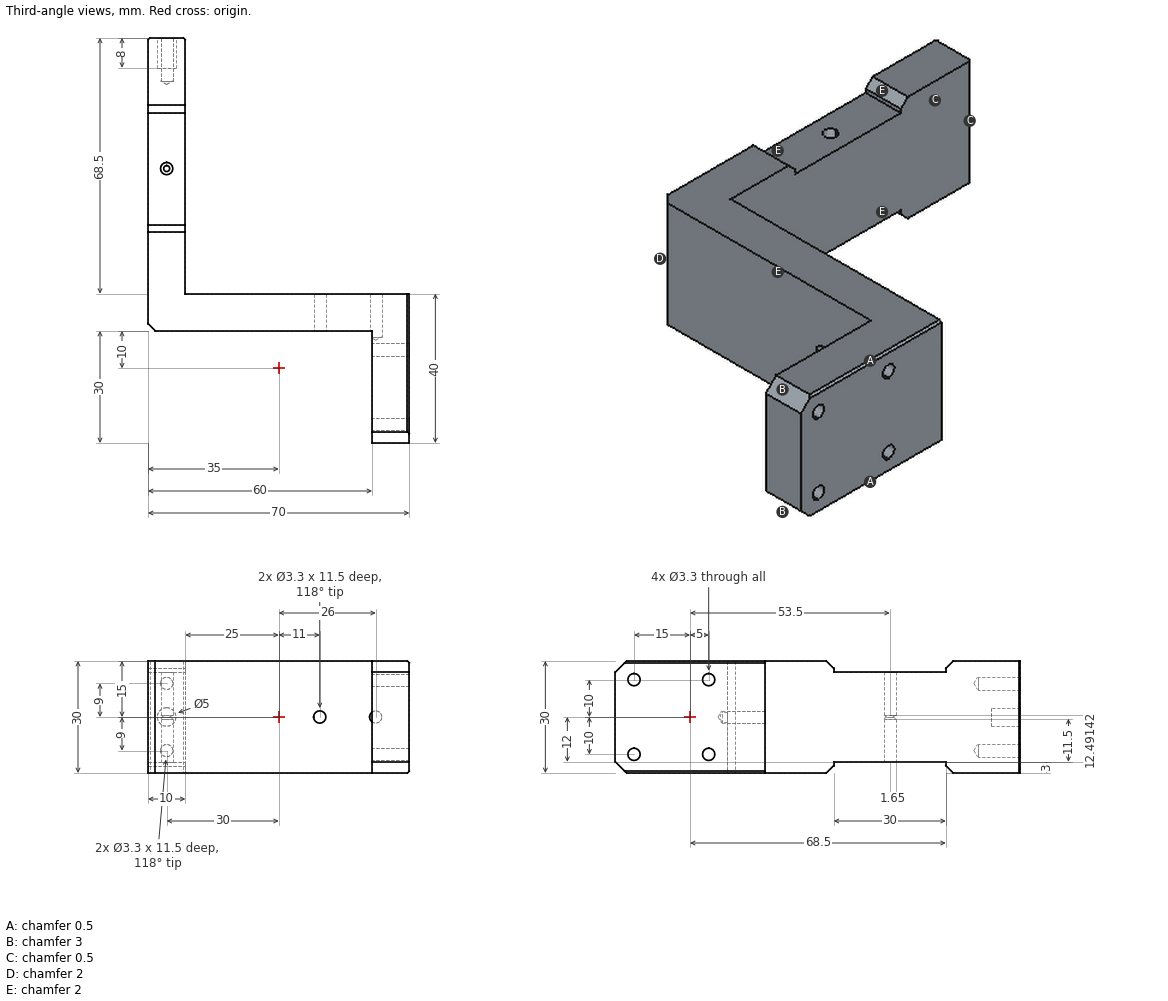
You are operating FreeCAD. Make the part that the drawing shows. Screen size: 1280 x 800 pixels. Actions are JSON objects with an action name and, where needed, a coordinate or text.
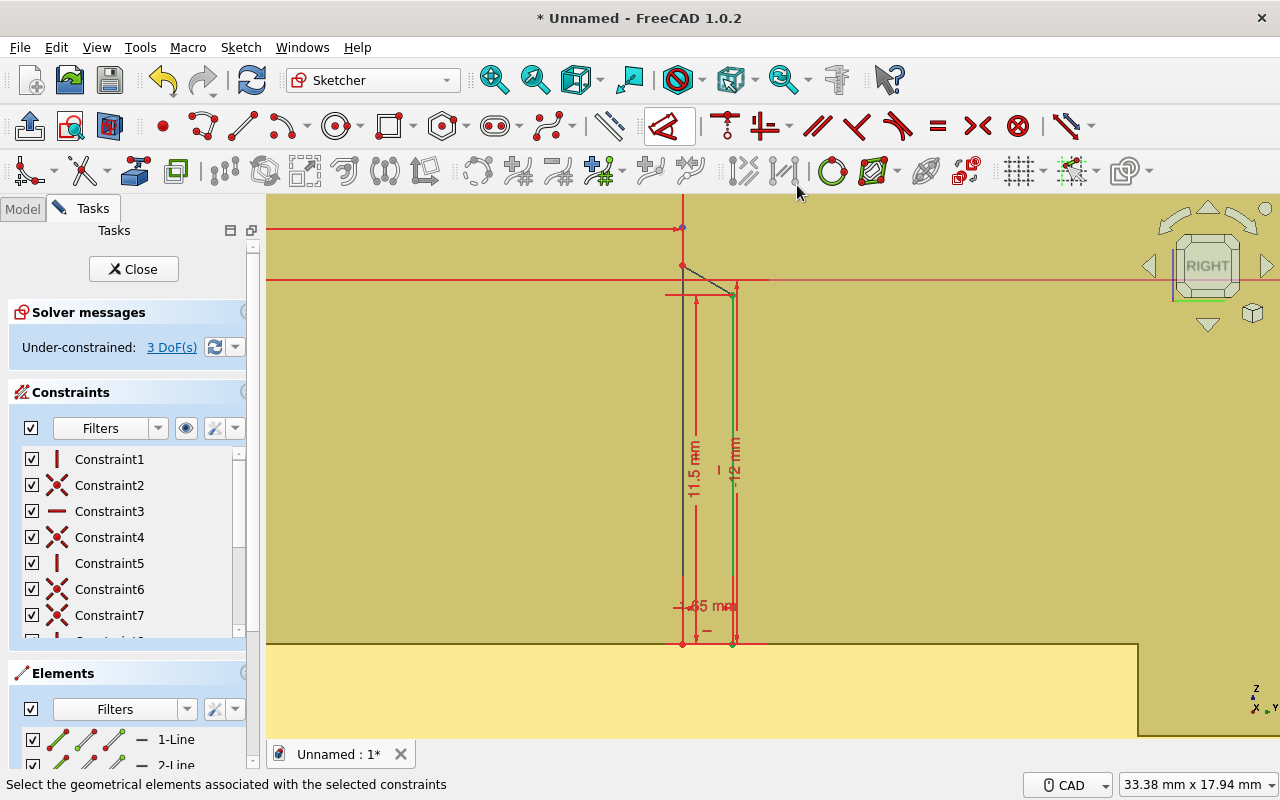
{"action": "left_click", "coordinate": [683, 379]}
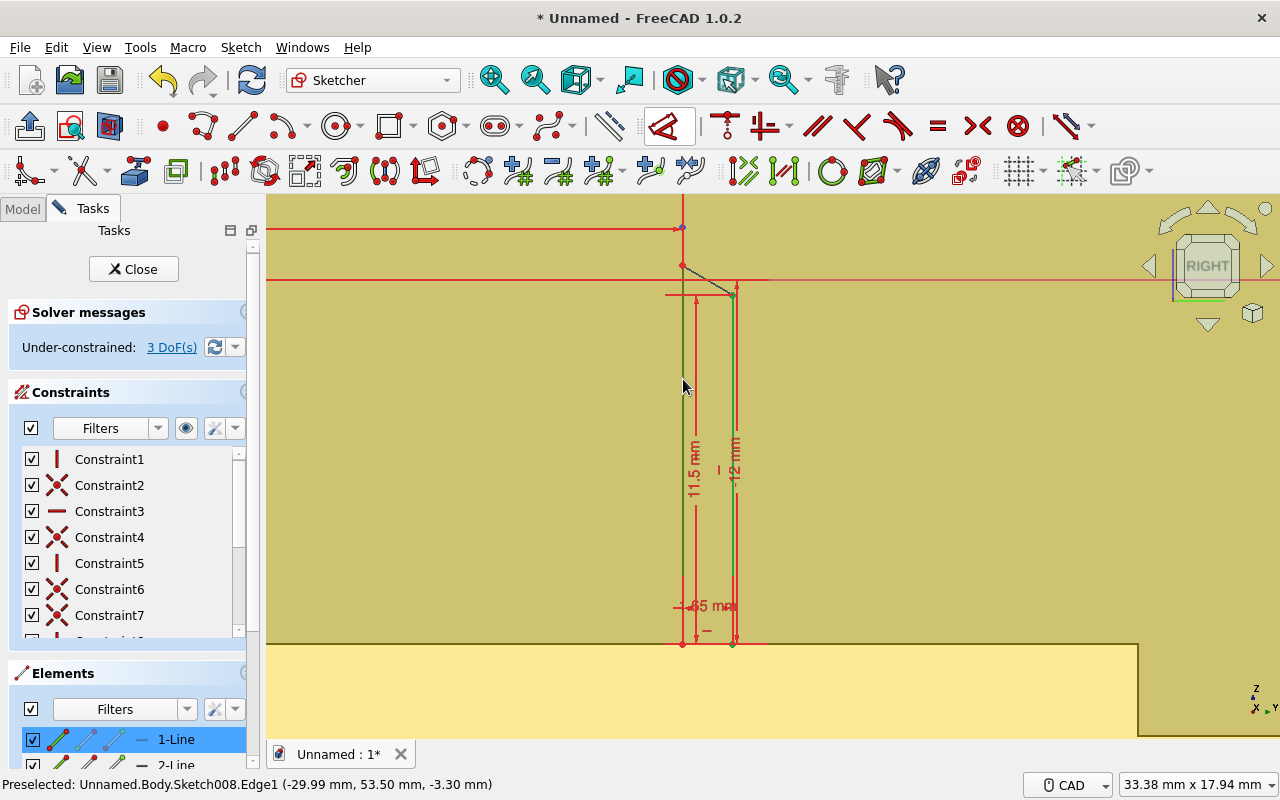
{"action": "key", "text": "i"}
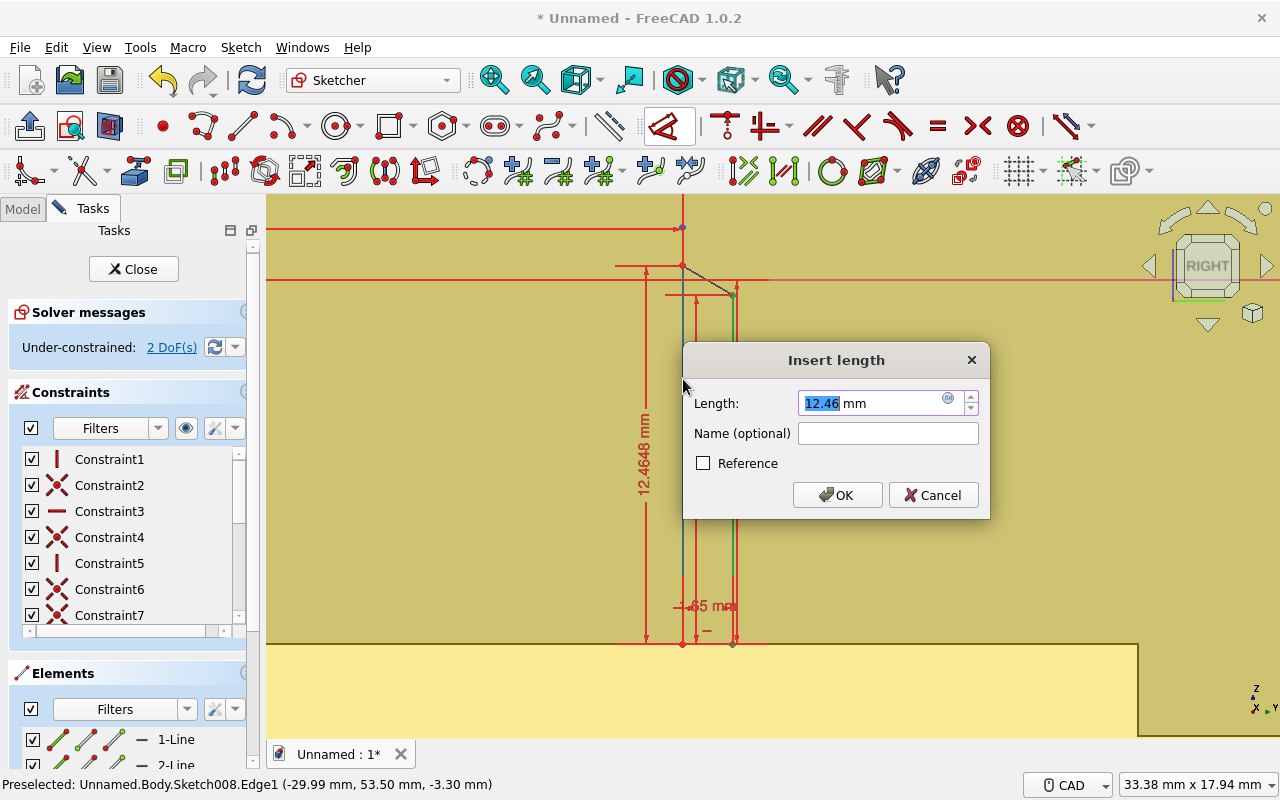
{"action": "type", "text": "12.49142"}
{"action": "key", "text": "Return"}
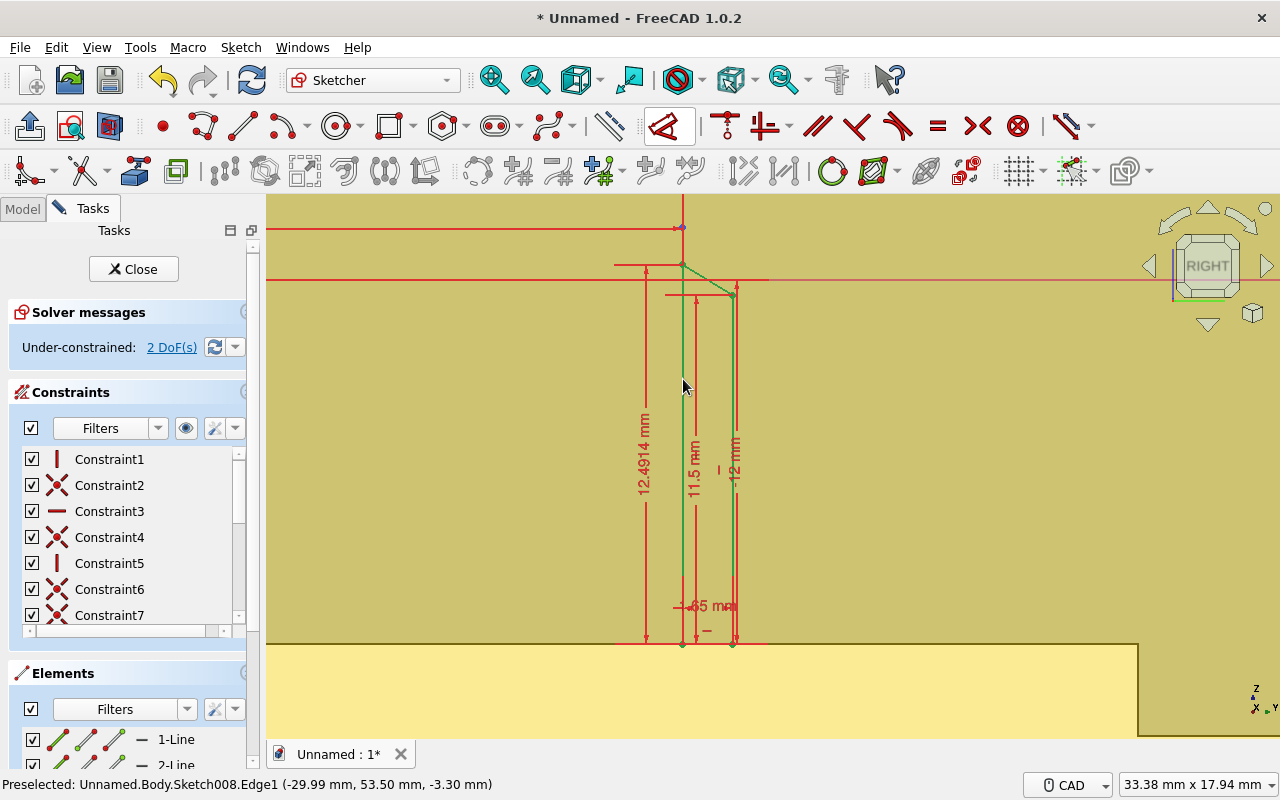
{"action": "left_click", "coordinate": [134, 269]}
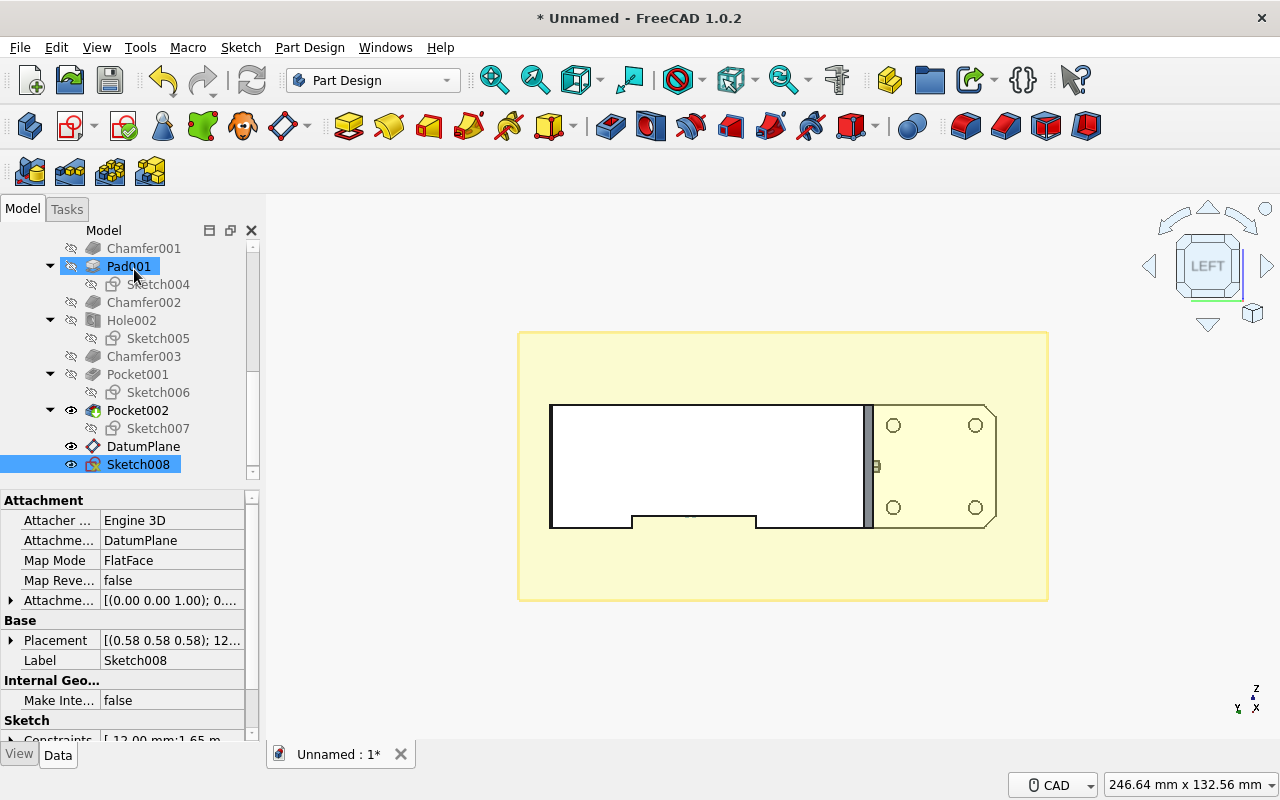
{"action": "left_click", "coordinate": [692, 126]}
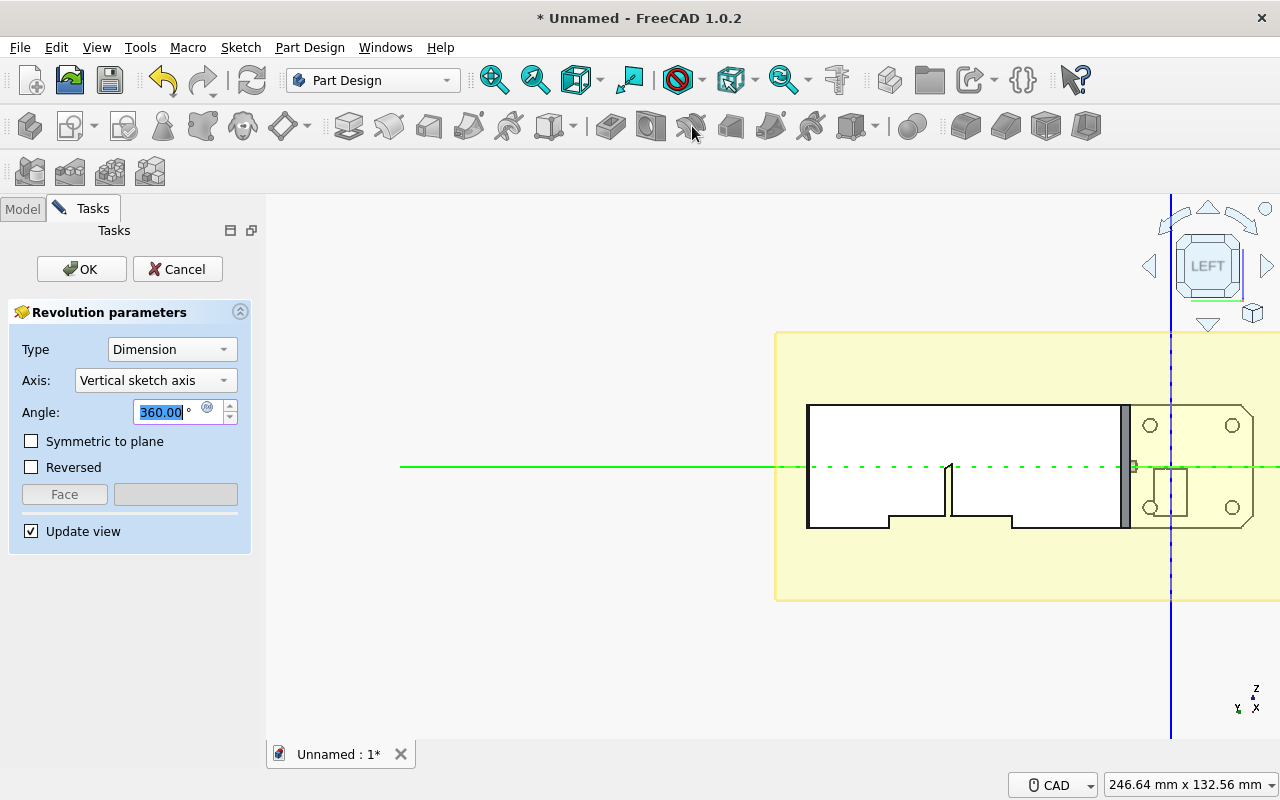
{"action": "left_click", "coordinate": [156, 380]}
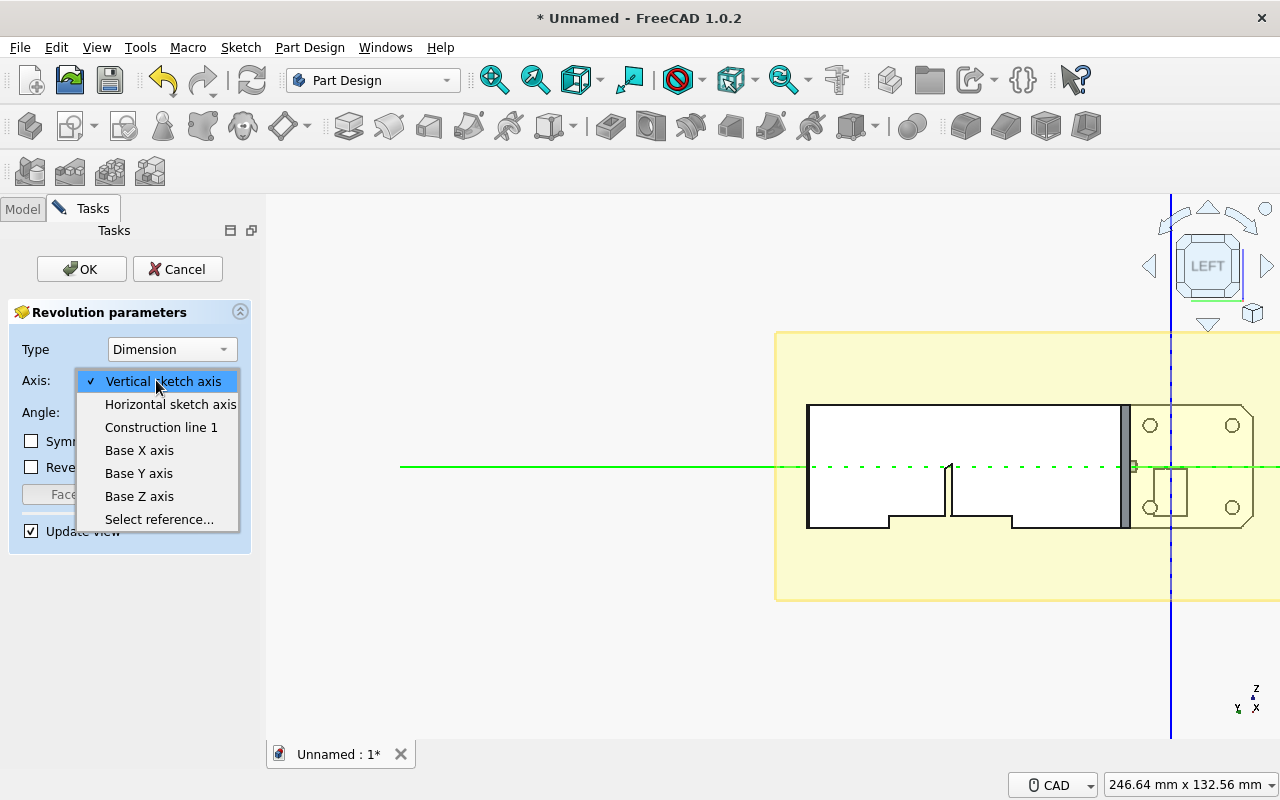
{"action": "left_click", "coordinate": [156, 428]}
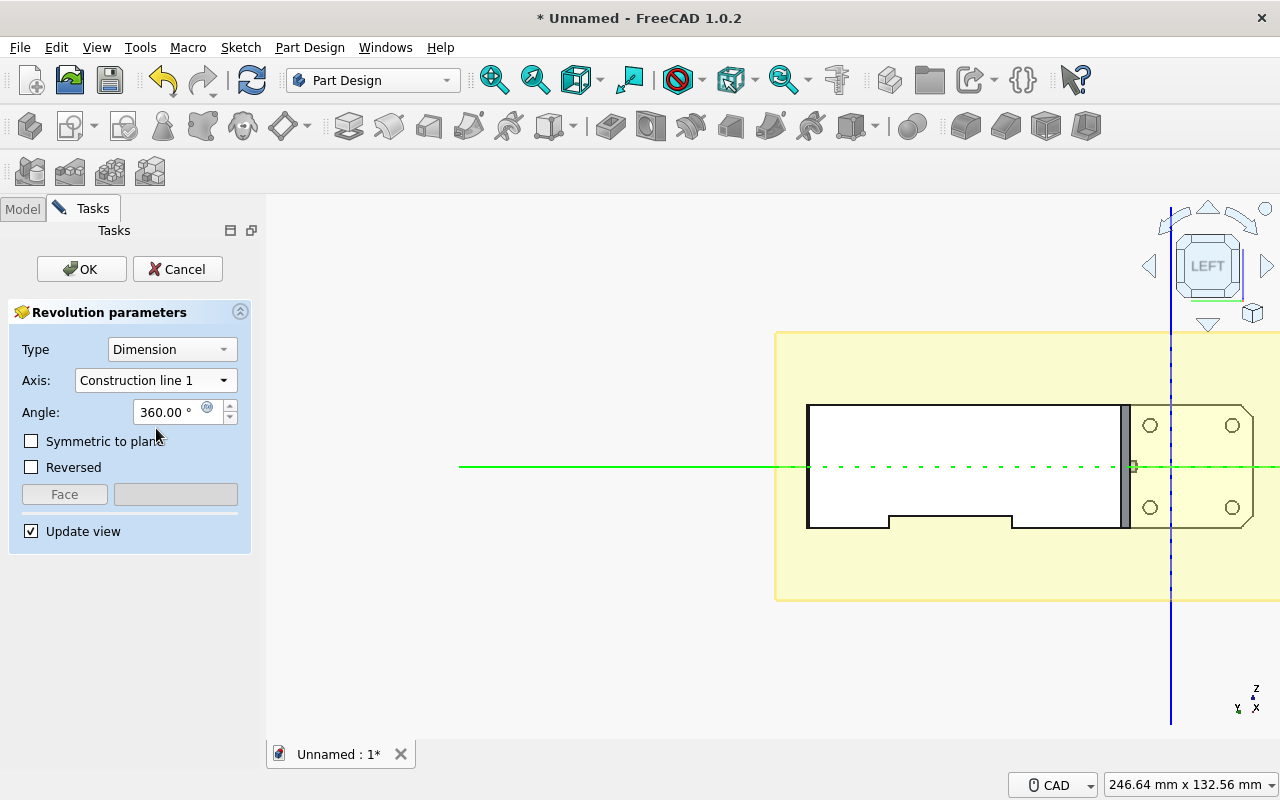
{"action": "left_click", "coordinate": [82, 269]}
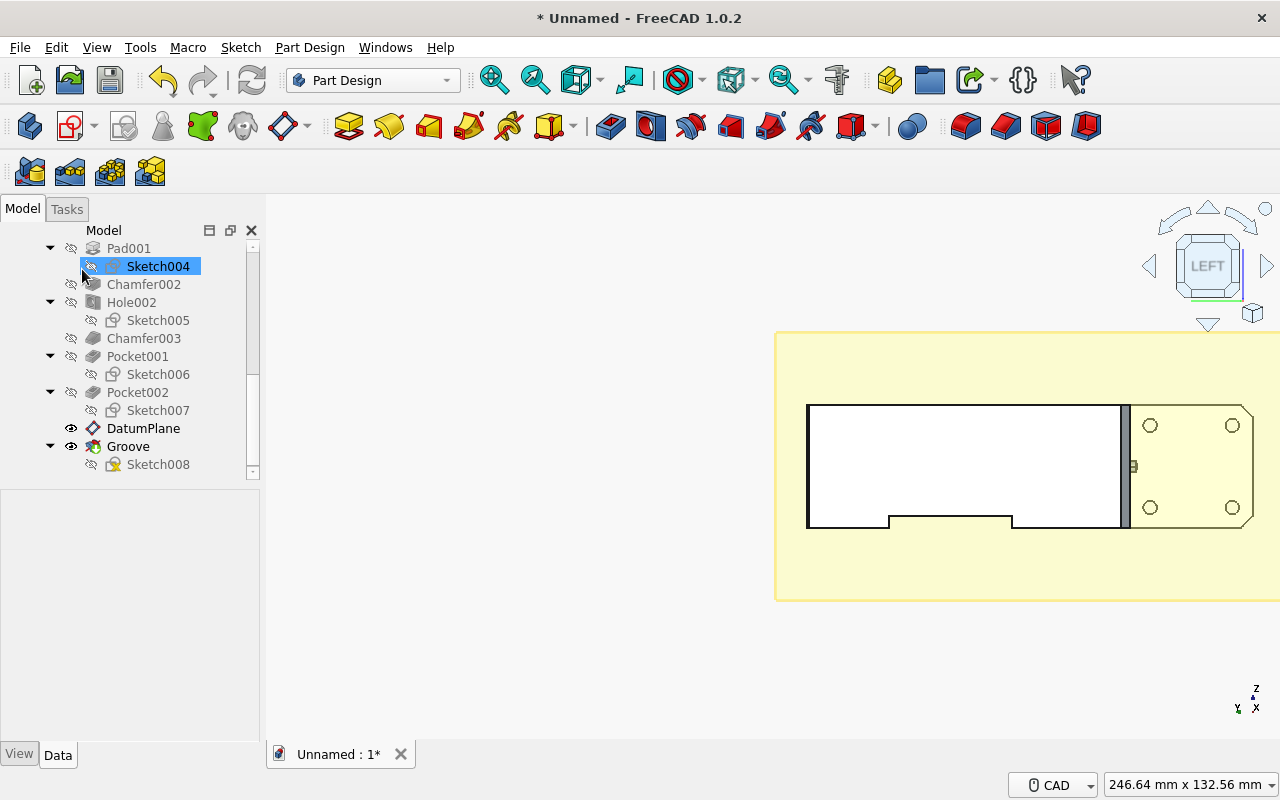
{"action": "left_click", "coordinate": [116, 428]}
{"action": "key", "text": "space"}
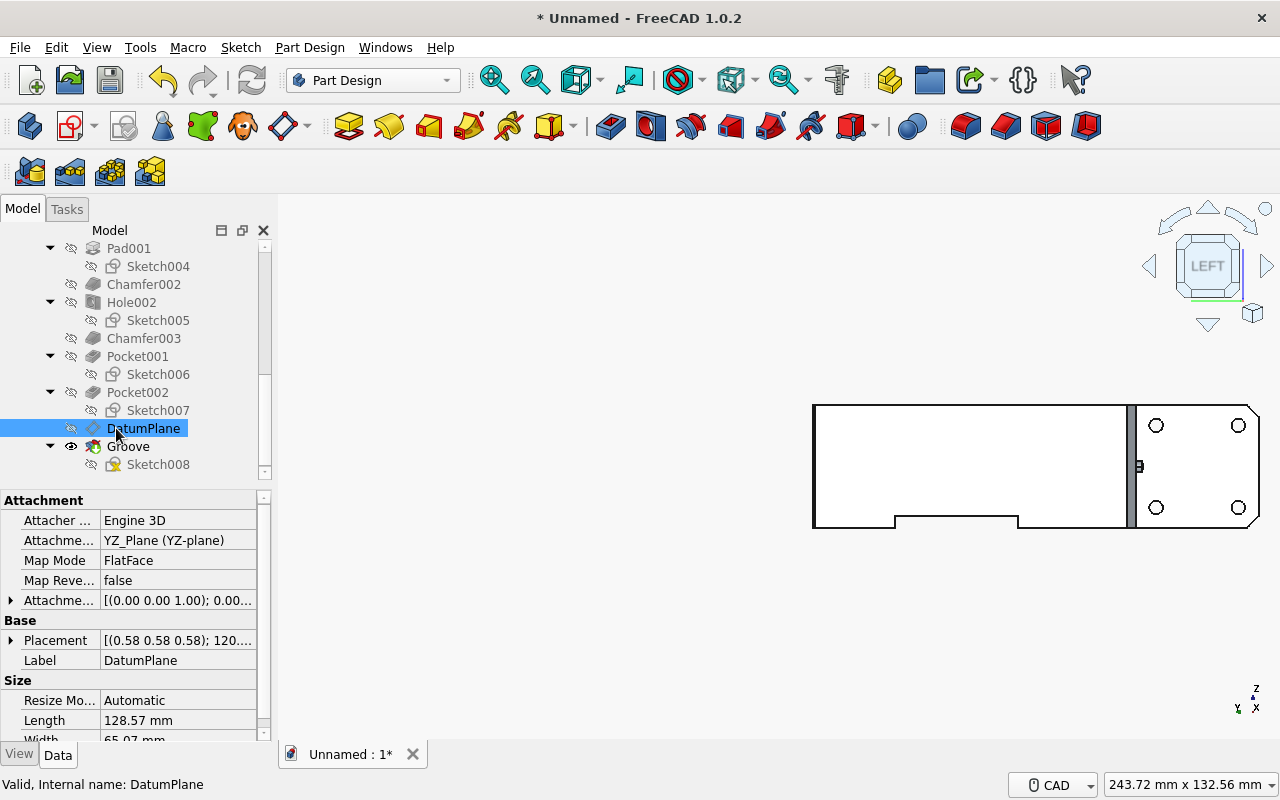
{"action": "key", "text": "v f"}